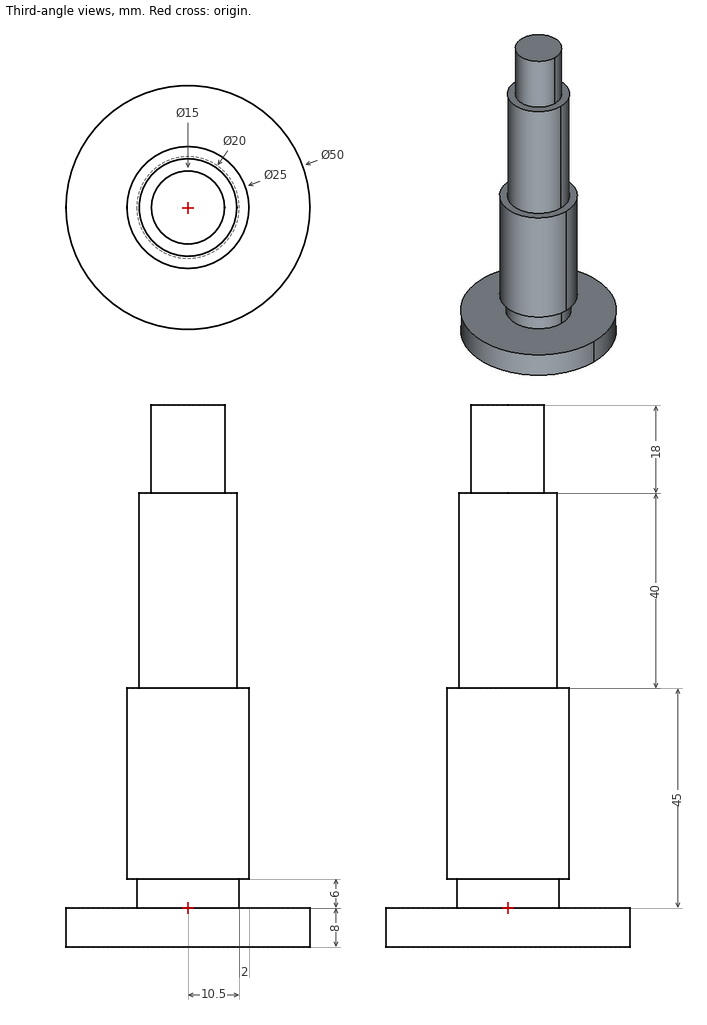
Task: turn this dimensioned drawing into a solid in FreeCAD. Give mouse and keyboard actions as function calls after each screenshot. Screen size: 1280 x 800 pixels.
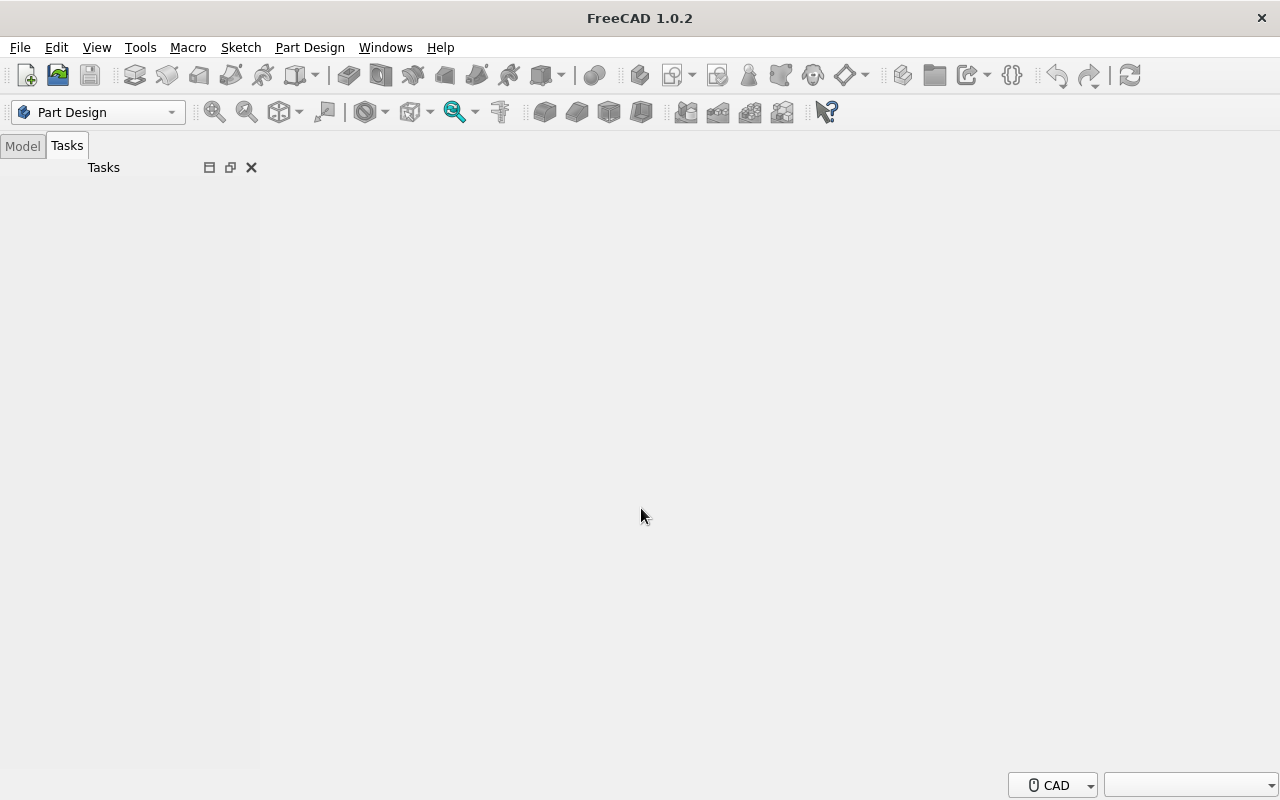
key(ctrl+n)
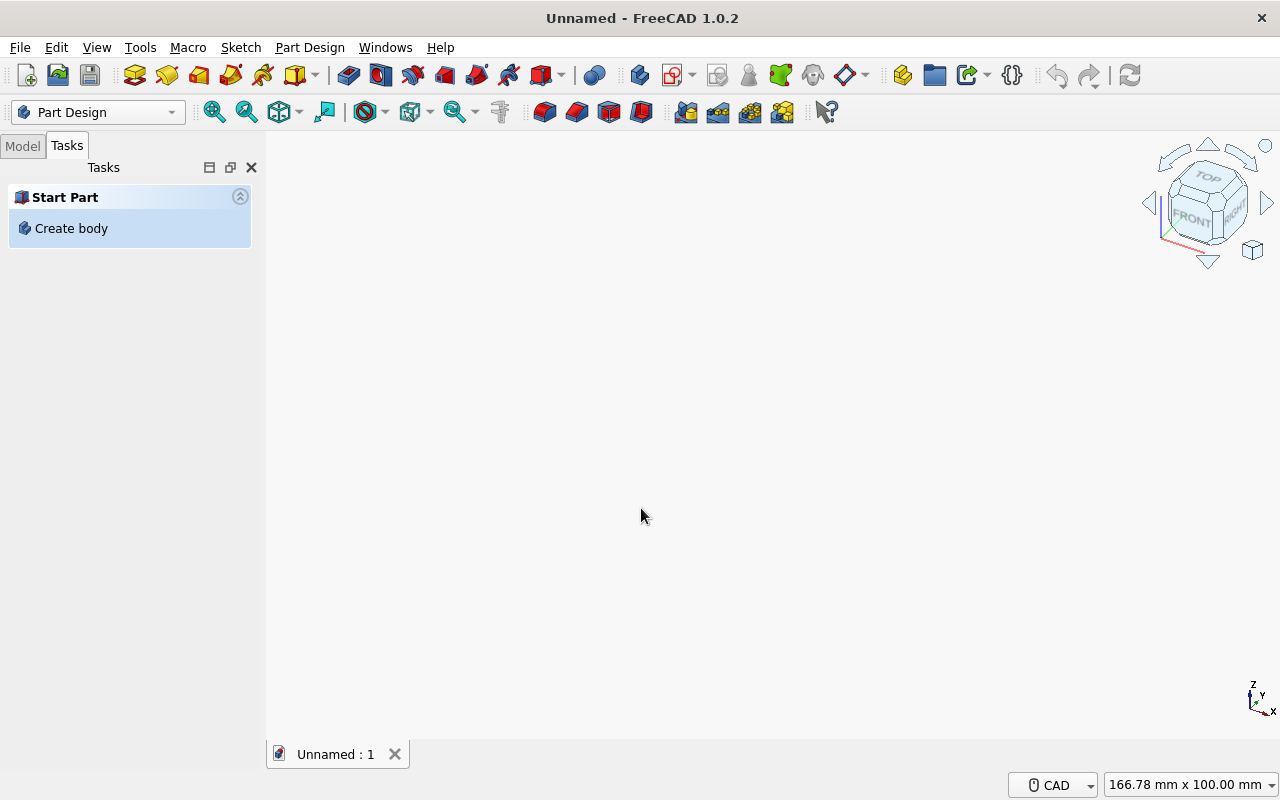
click(672, 76)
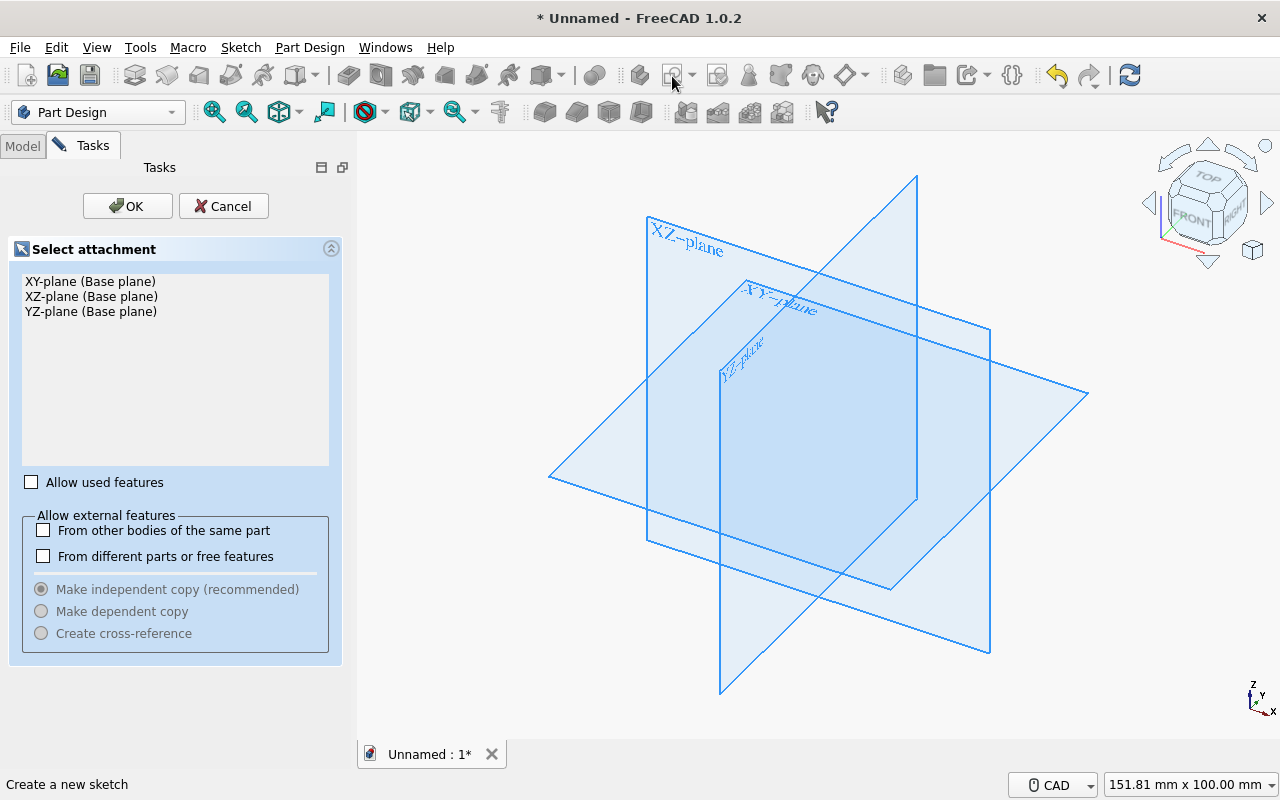
click(82, 282)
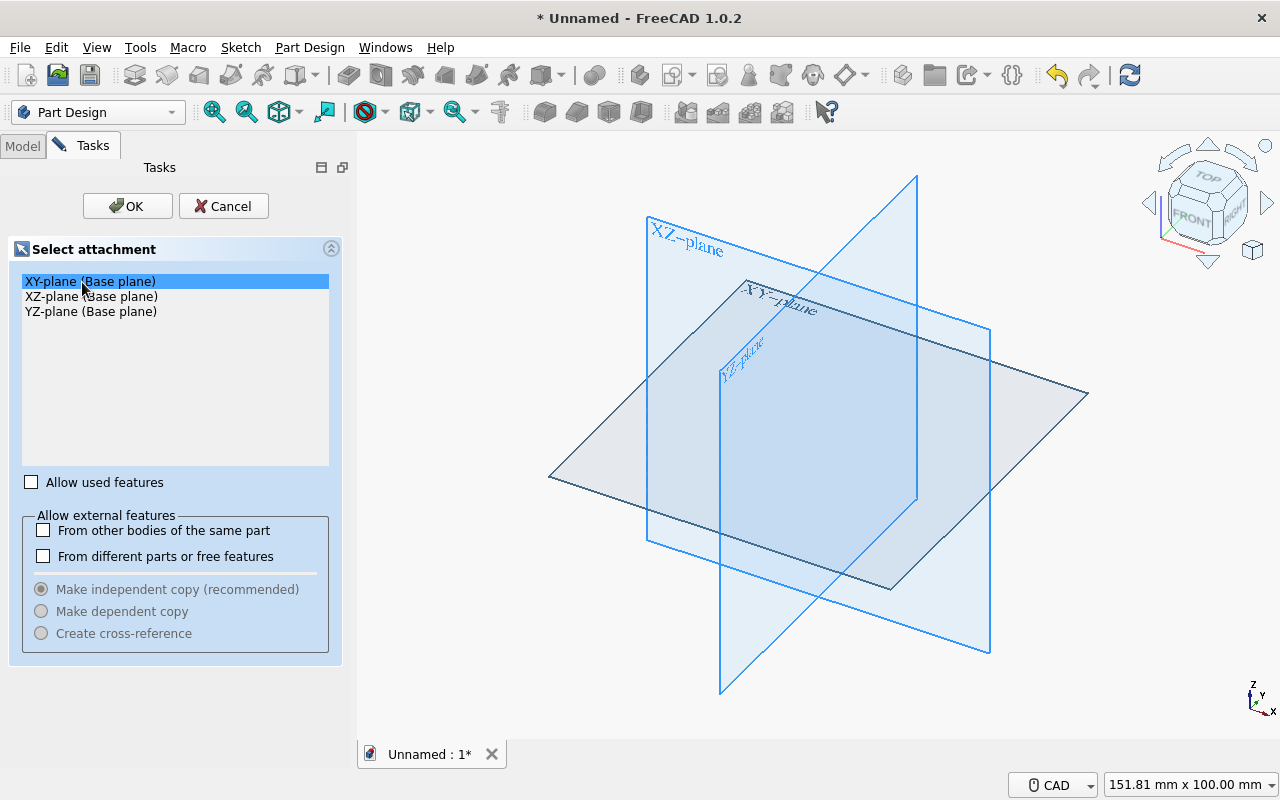
click(128, 206)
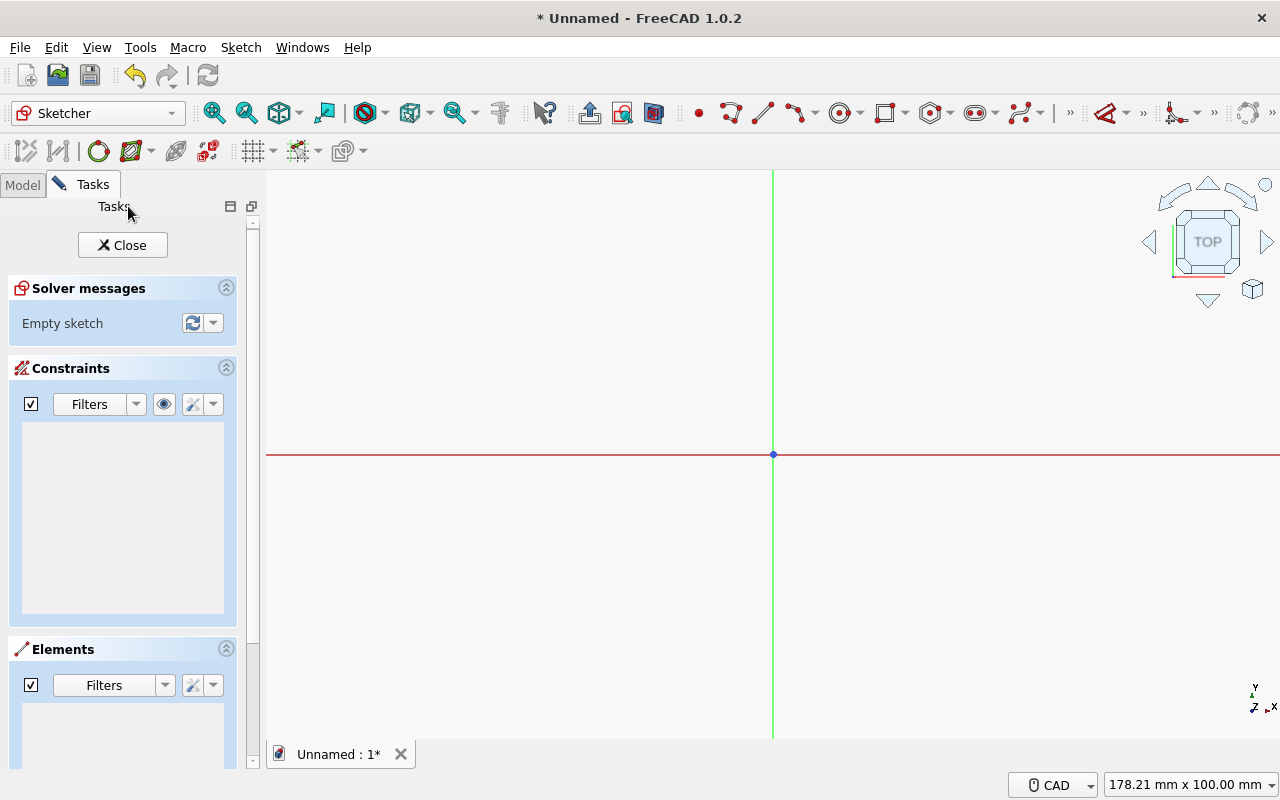
scroll(813, 454, up, 5)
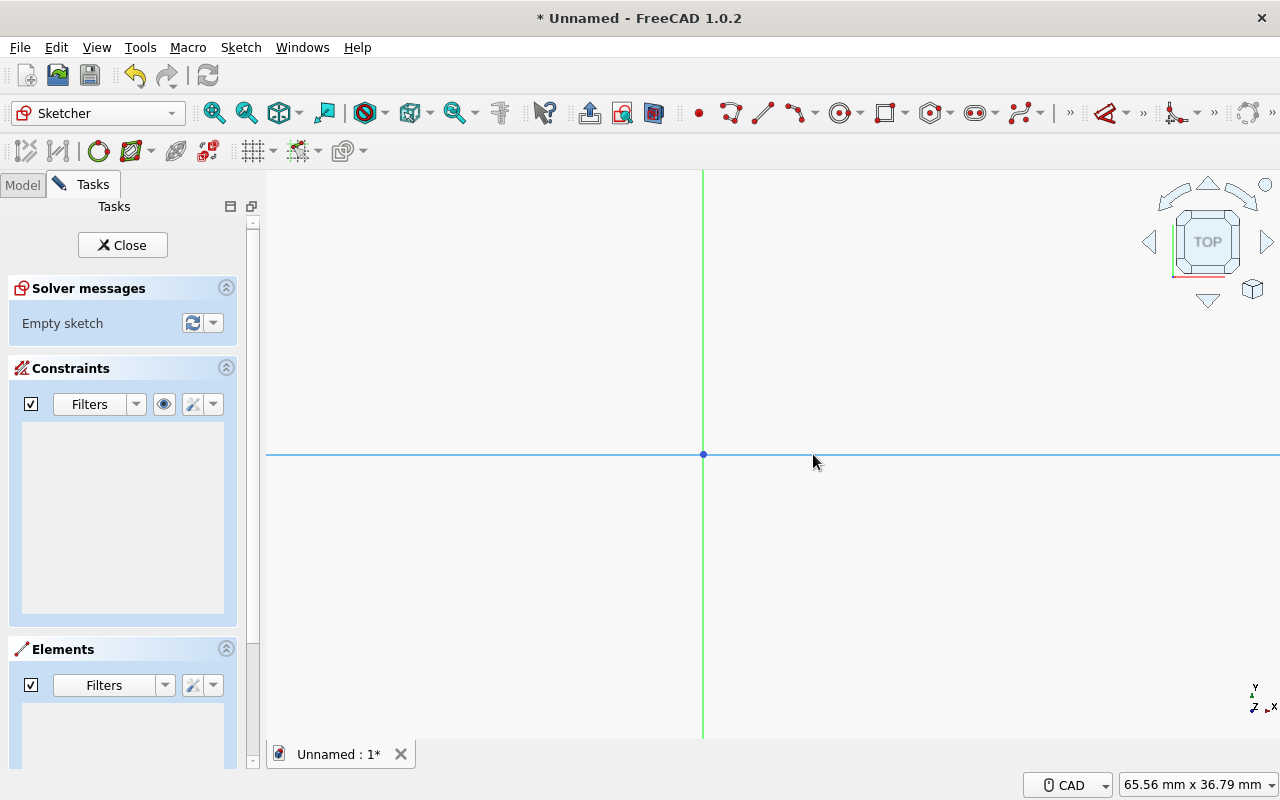
key(g)
key(c)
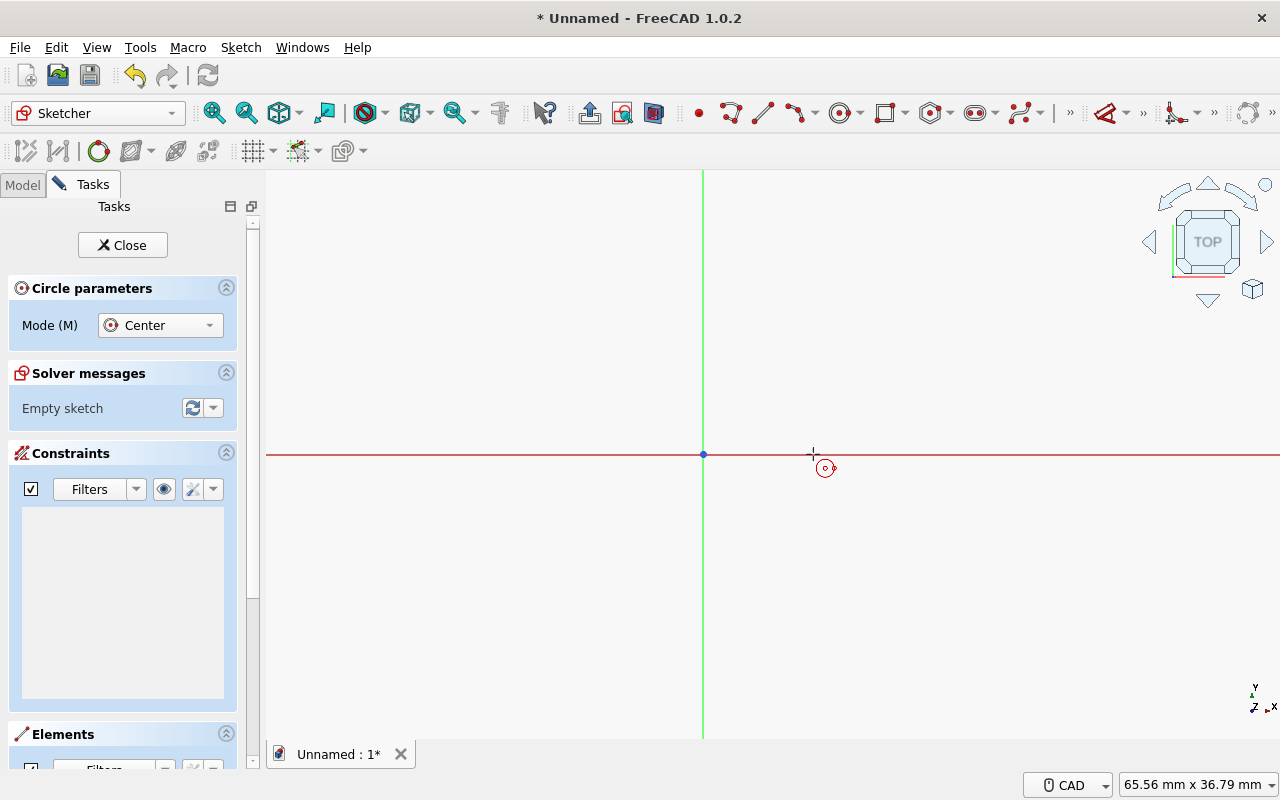
click(703, 454)
move(840, 318)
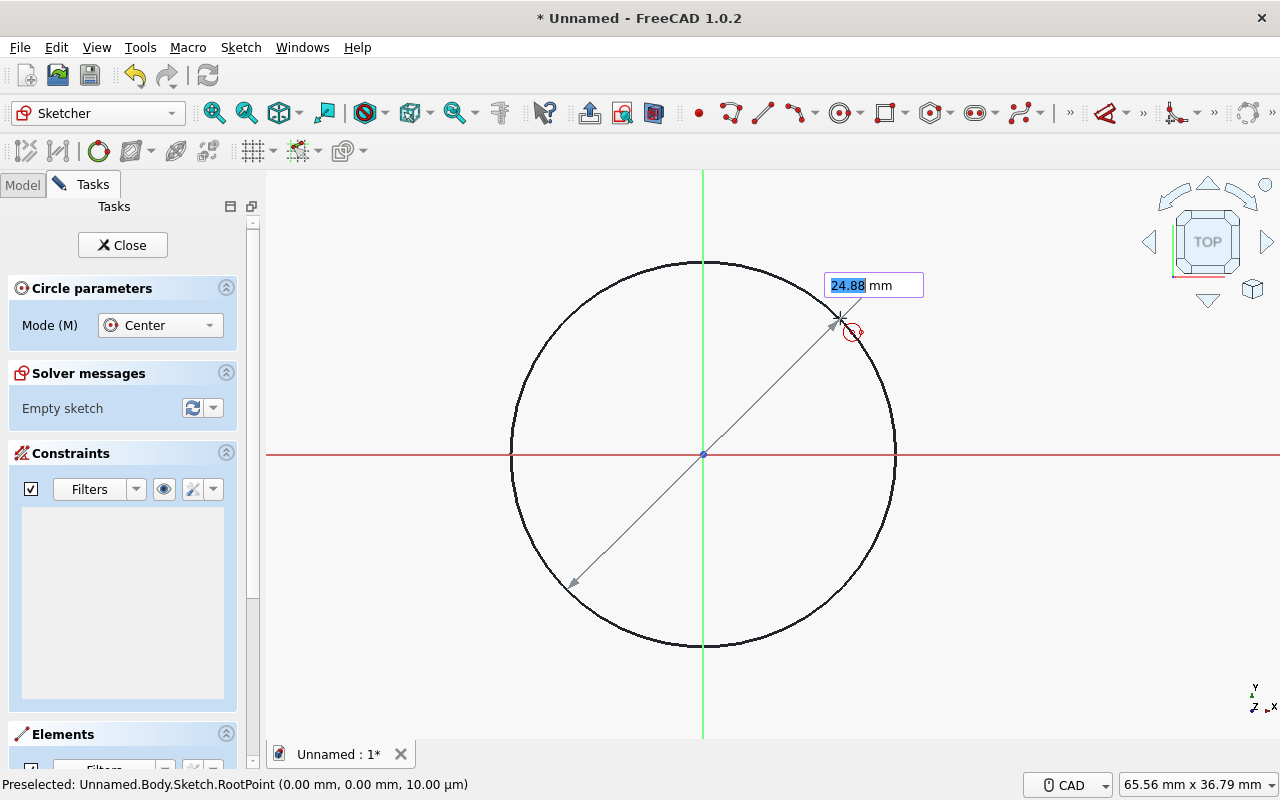
text(25)
key(Return)
key(Escape)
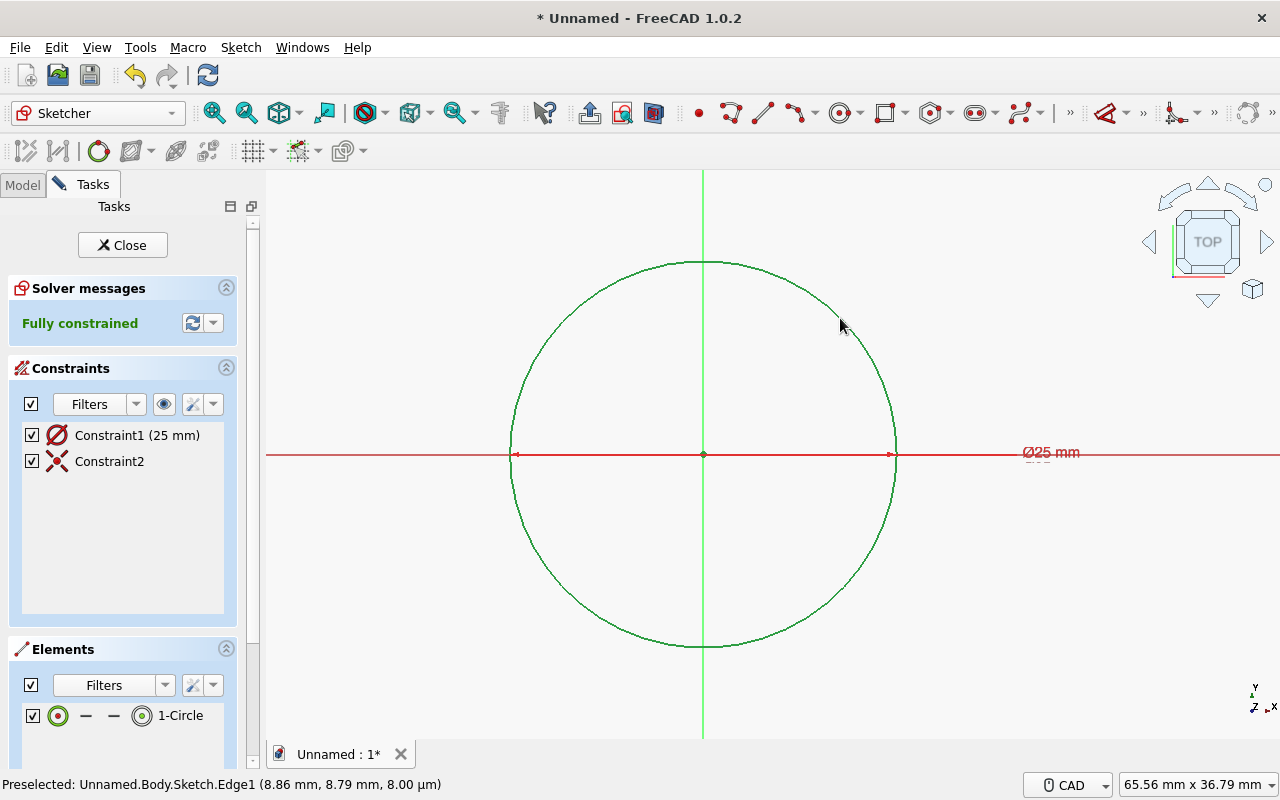
click(123, 245)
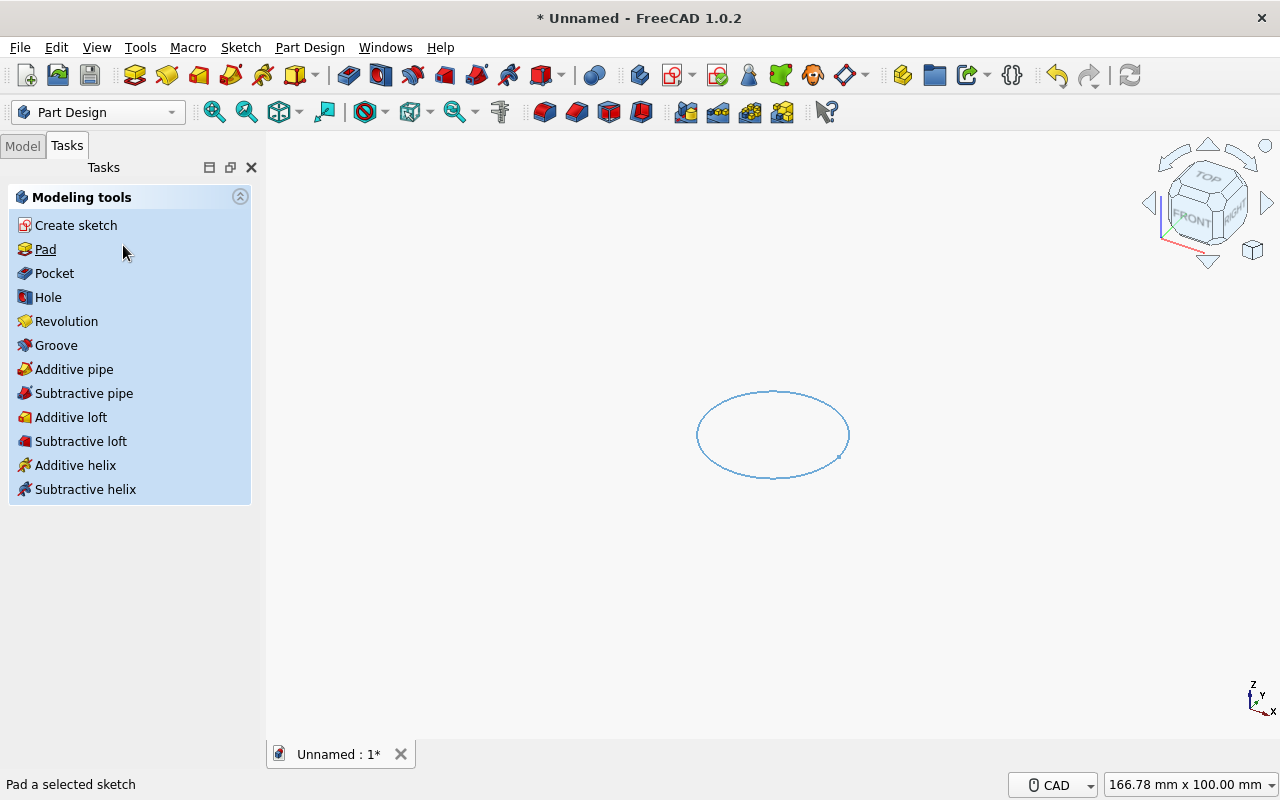
click(136, 76)